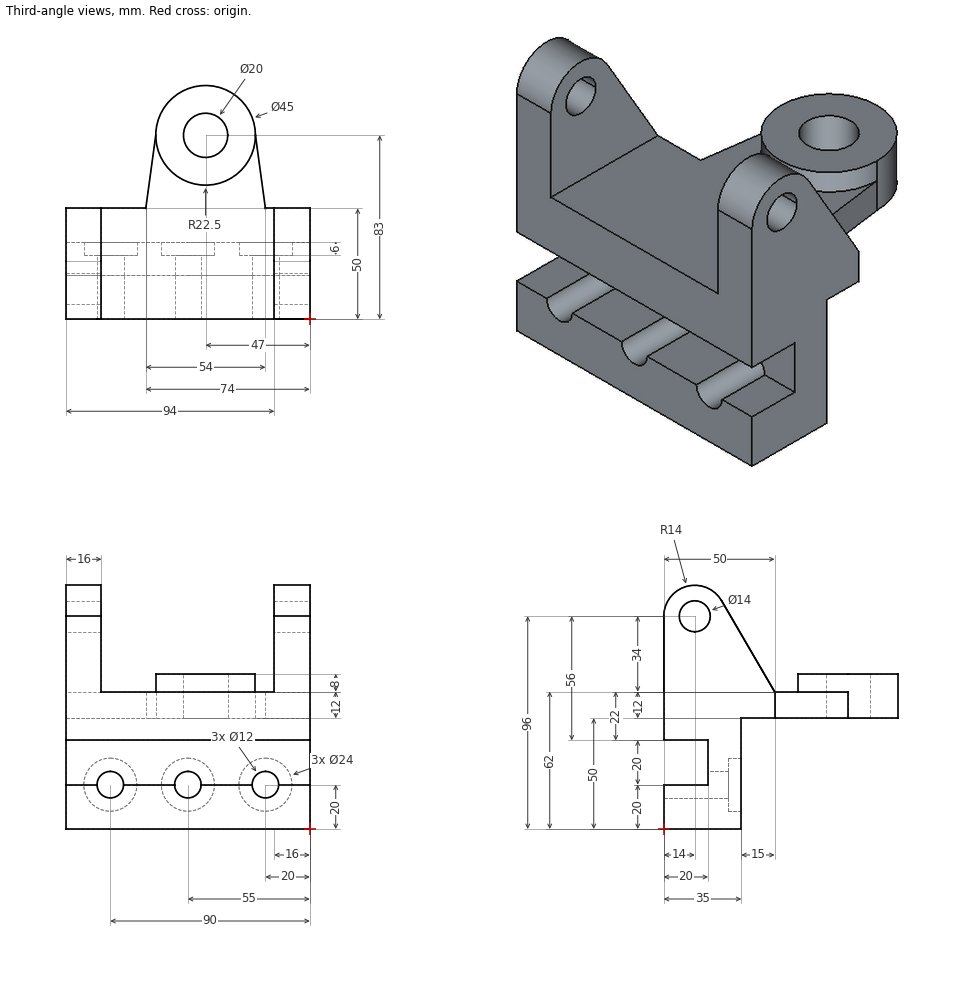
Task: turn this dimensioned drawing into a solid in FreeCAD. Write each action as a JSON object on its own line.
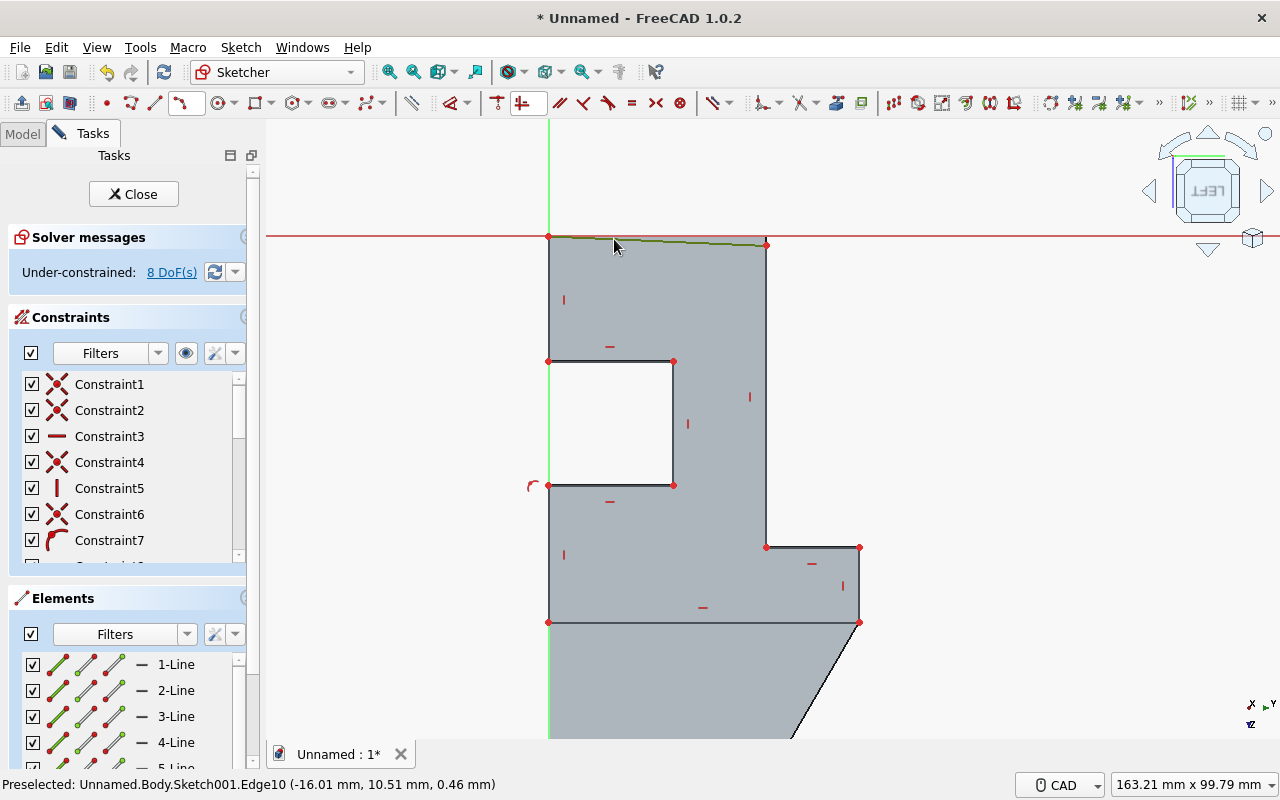
{"action": "left_click", "coordinate": [542, 104]}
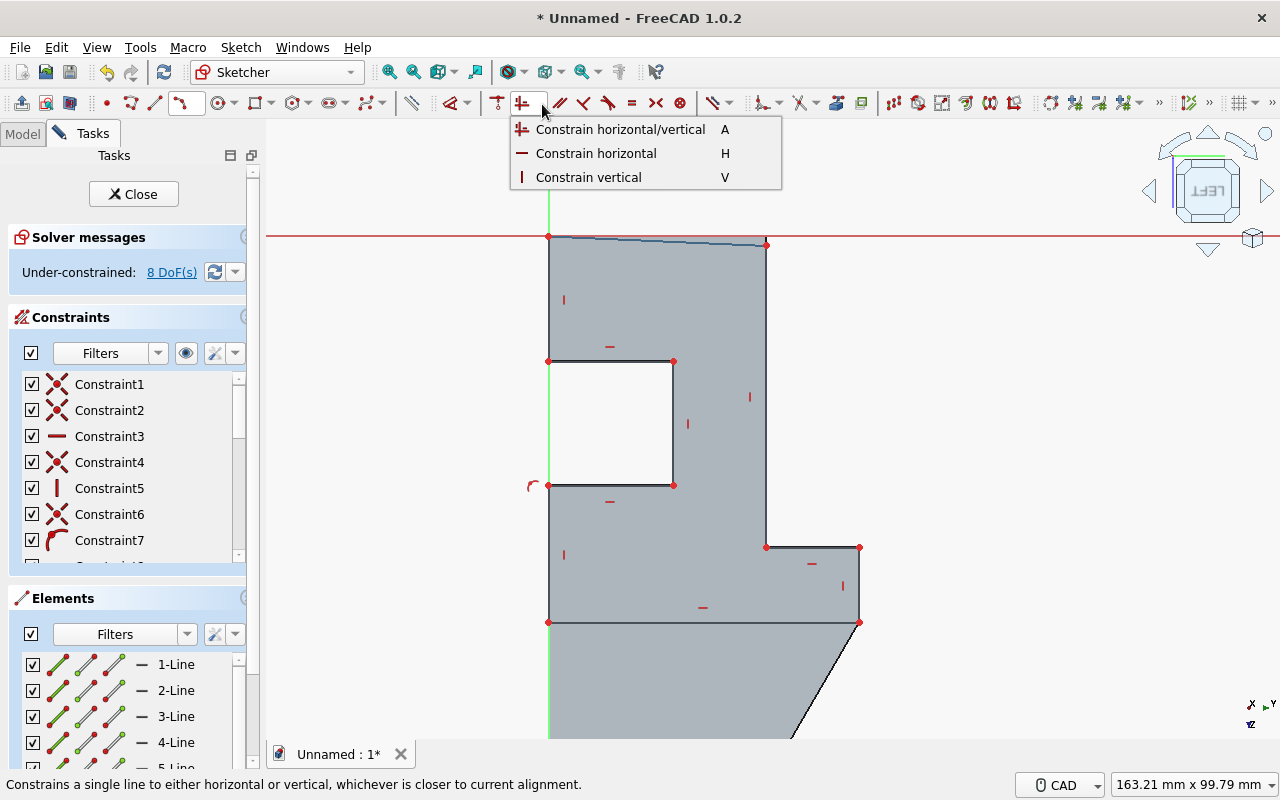
{"action": "left_click", "coordinate": [646, 153]}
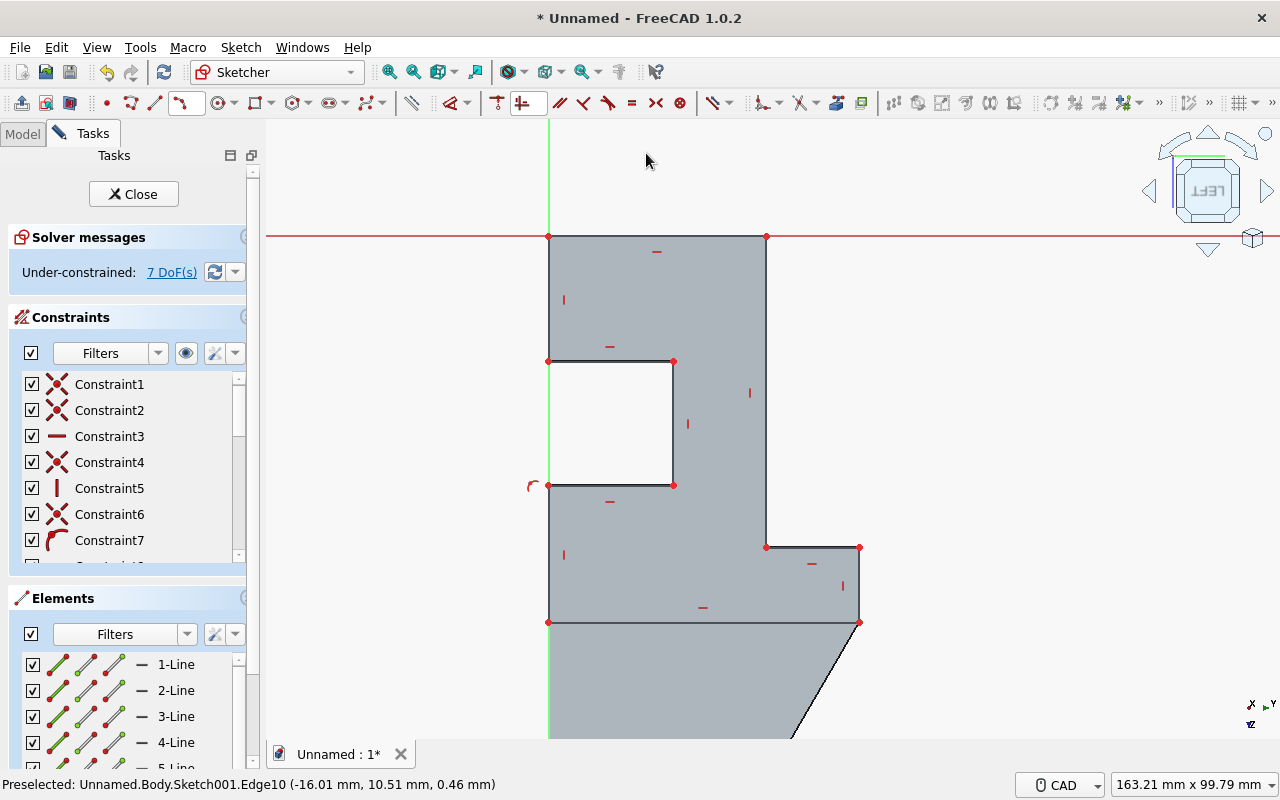
{"action": "left_click", "coordinate": [450, 104]}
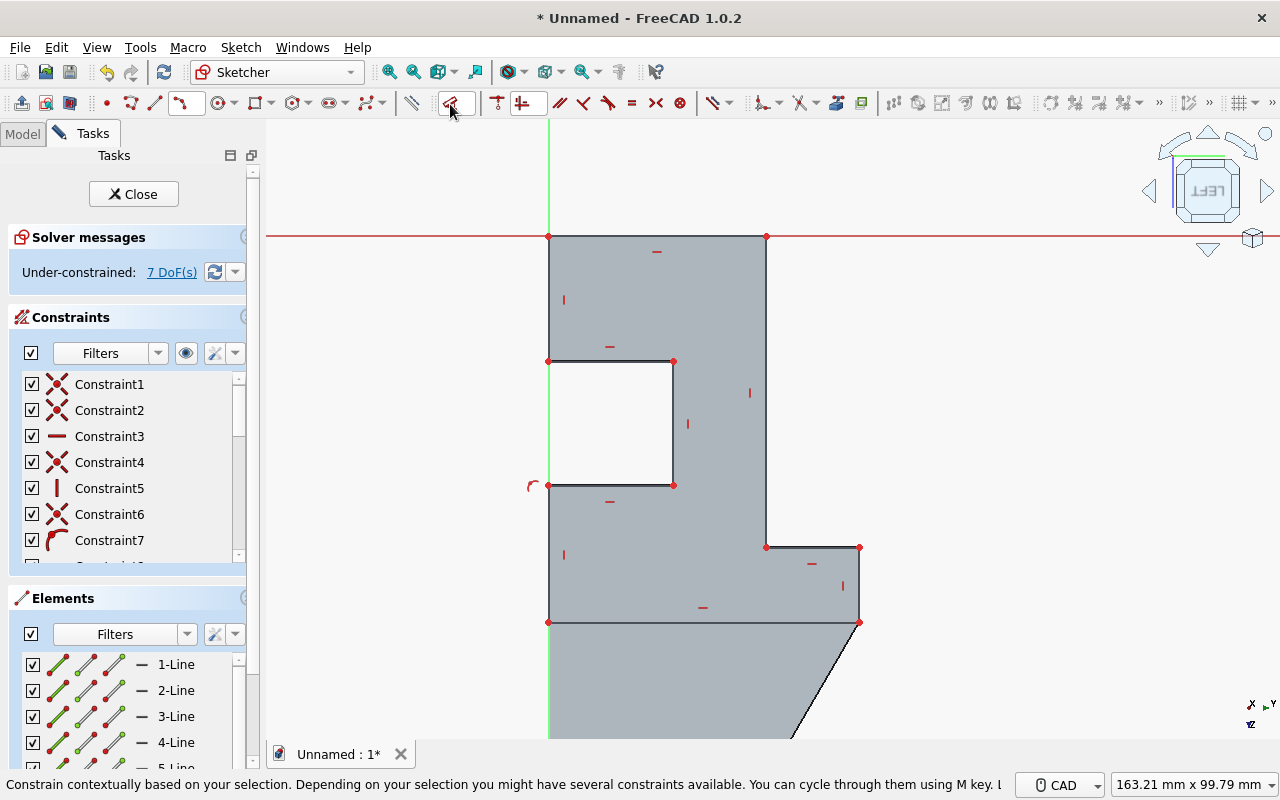
{"action": "left_click", "coordinate": [549, 274]}
{"action": "left_click", "coordinate": [515, 299]}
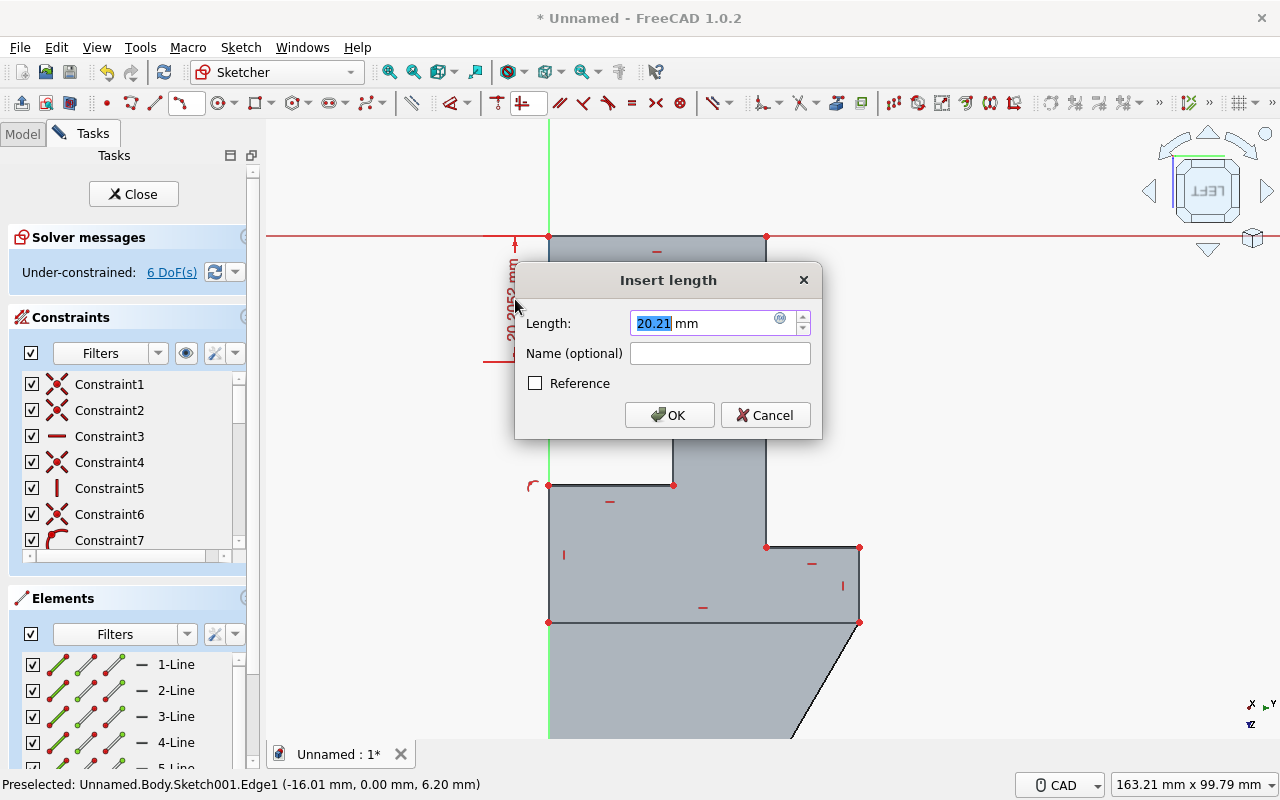
{"action": "type", "text": "20"}
{"action": "key", "text": "Return"}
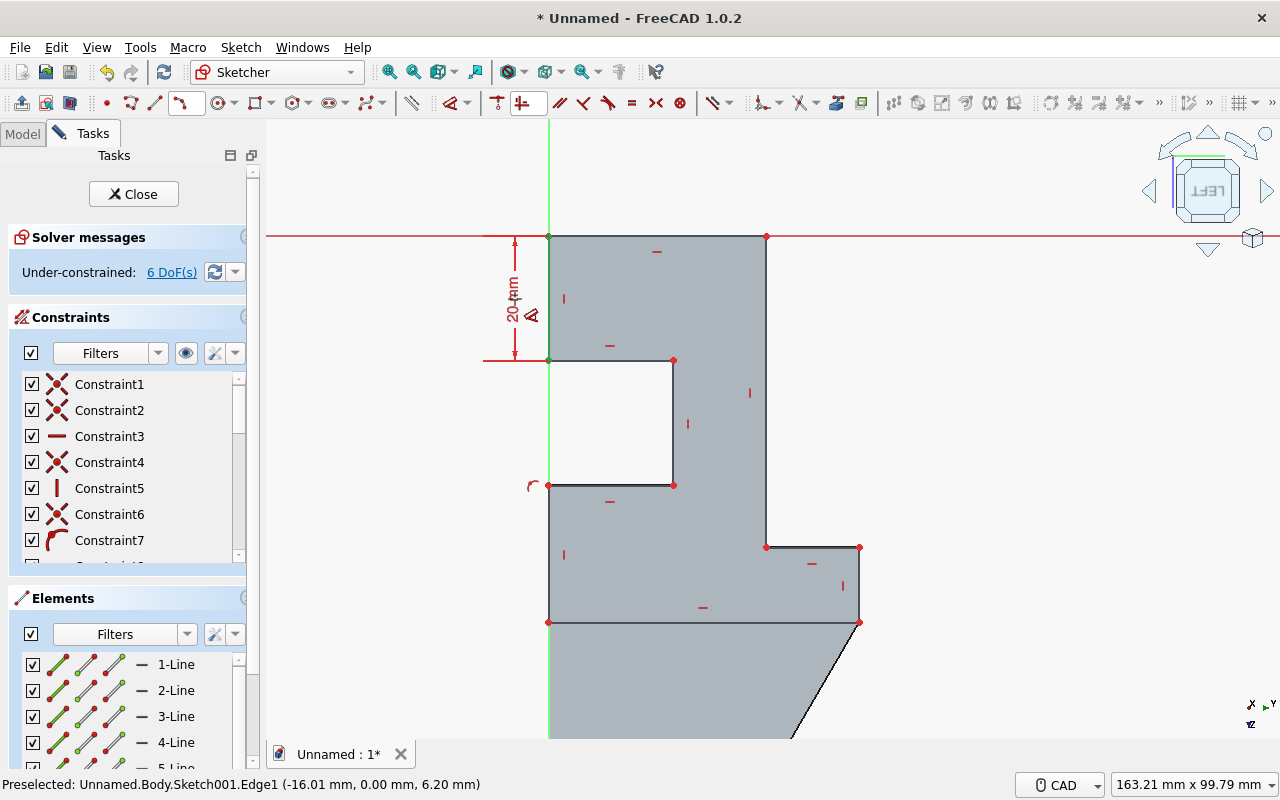
{"action": "left_click", "coordinate": [586, 361]}
{"action": "left_click", "coordinate": [611, 327]}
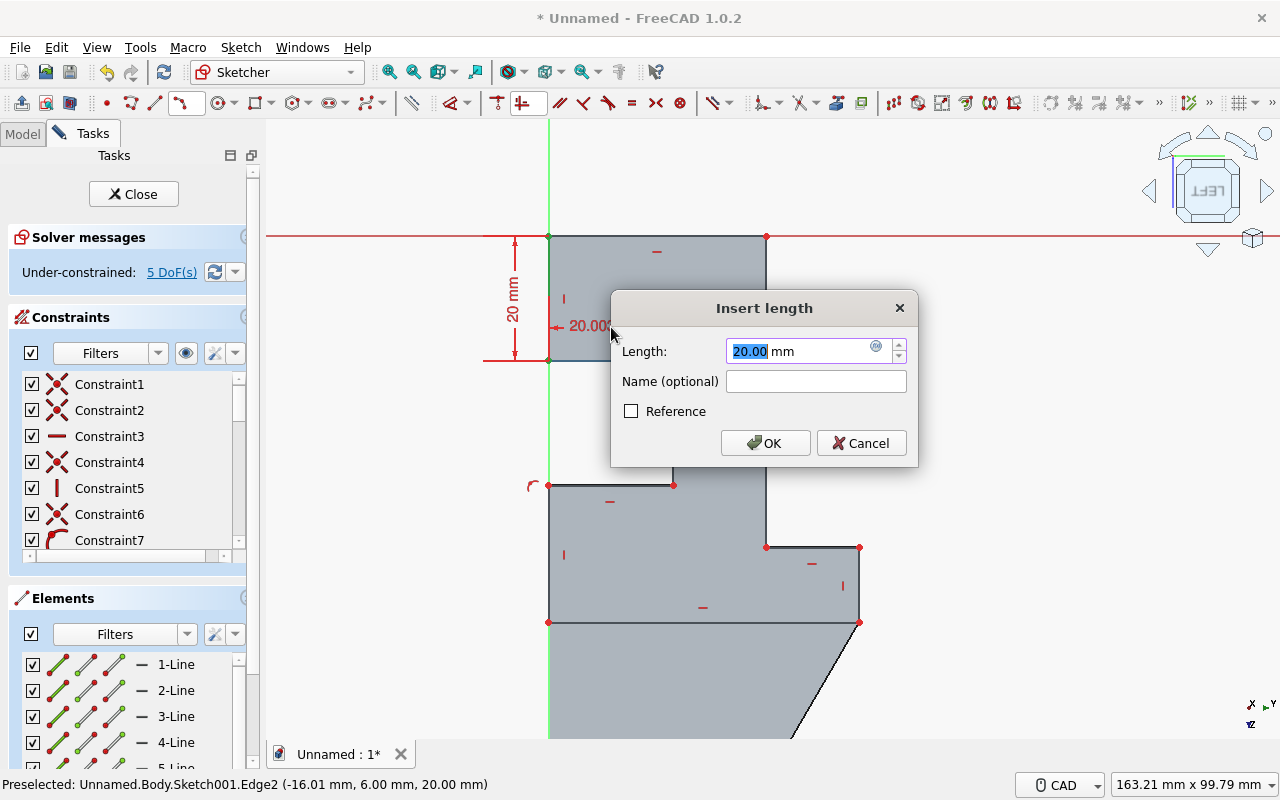
{"action": "type", "text": "20"}
{"action": "key", "text": "Return"}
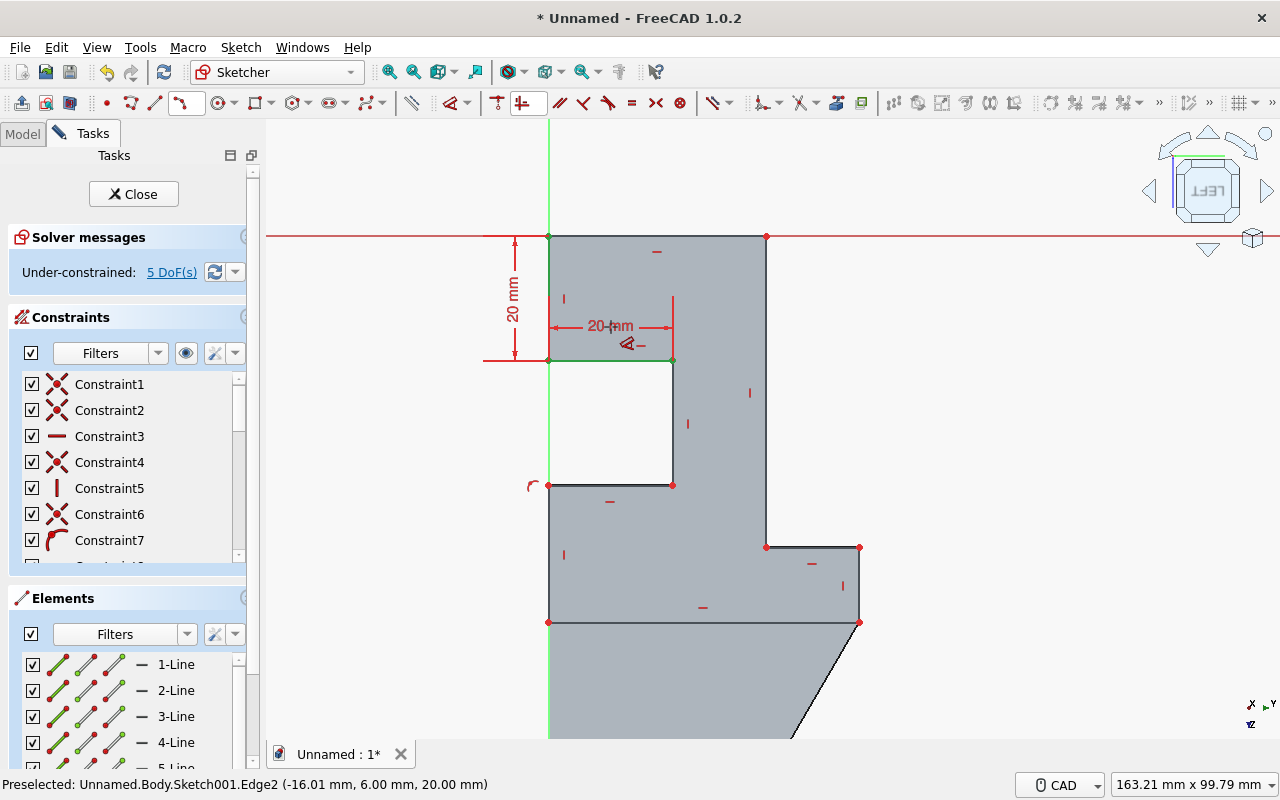
{"action": "left_click", "coordinate": [673, 398]}
{"action": "left_click", "coordinate": [639, 423]}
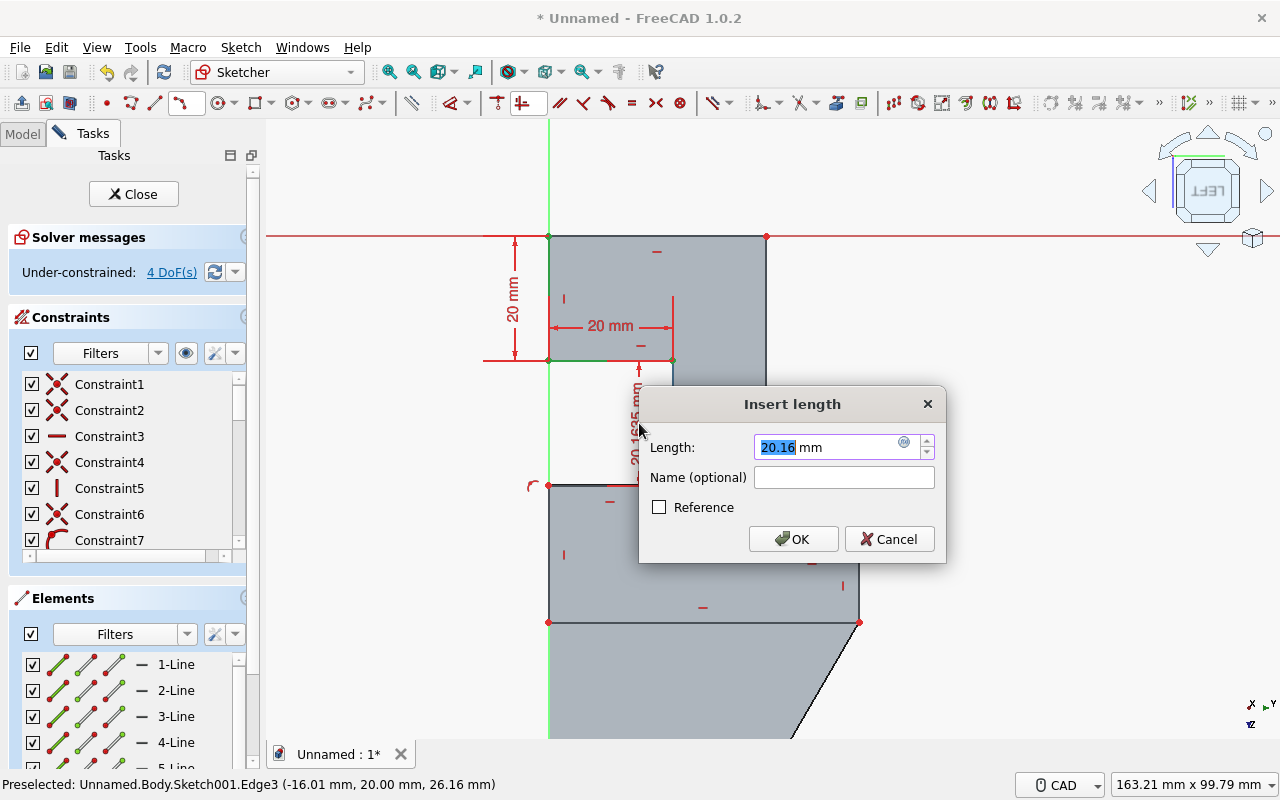
{"action": "type", "text": "20"}
{"action": "key", "text": "Return"}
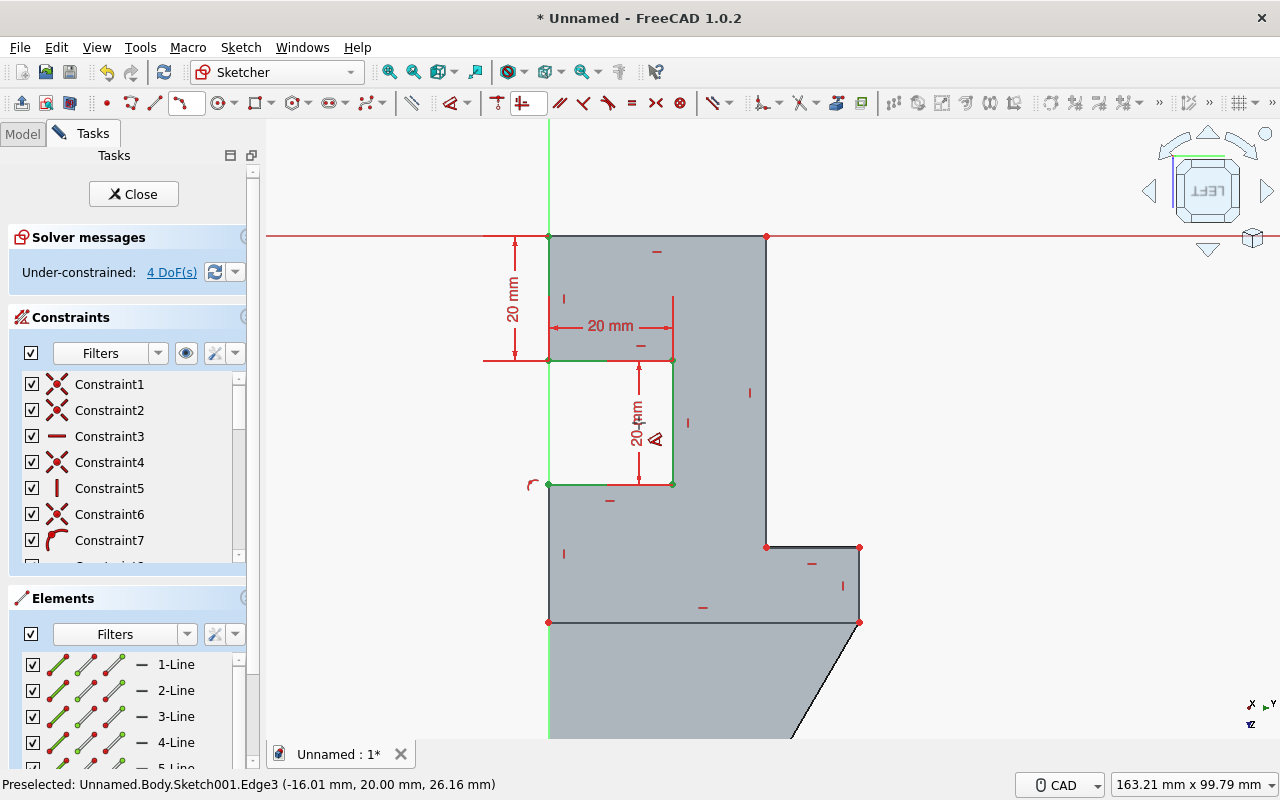
{"action": "left_click", "coordinate": [549, 526]}
{"action": "left_click", "coordinate": [515, 554]}